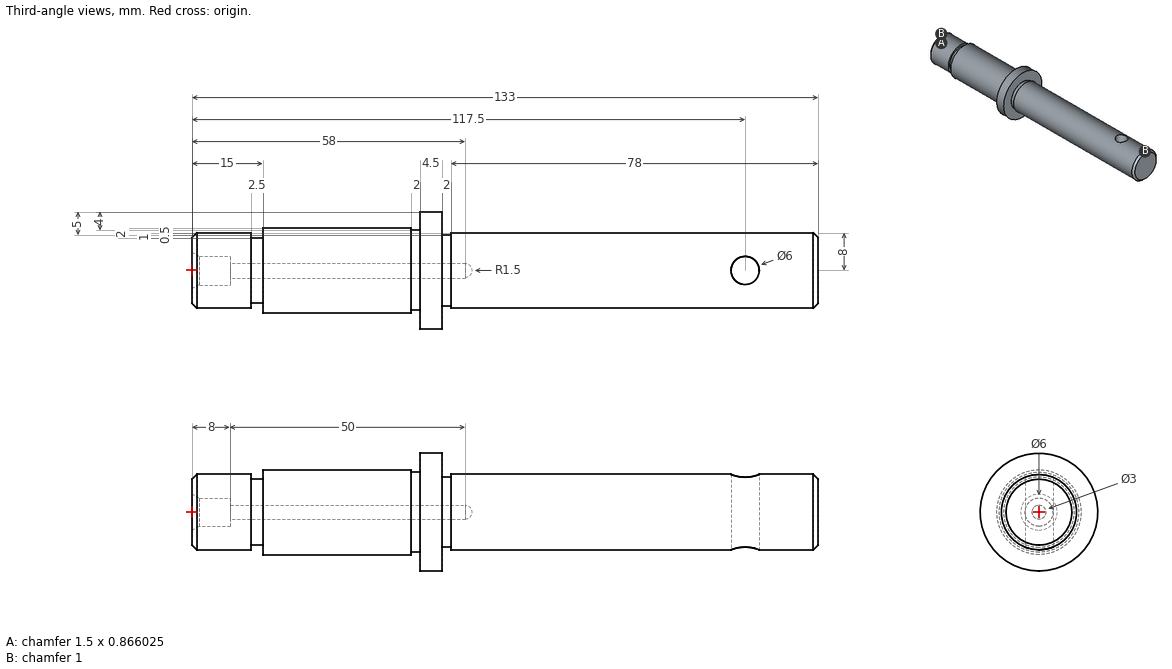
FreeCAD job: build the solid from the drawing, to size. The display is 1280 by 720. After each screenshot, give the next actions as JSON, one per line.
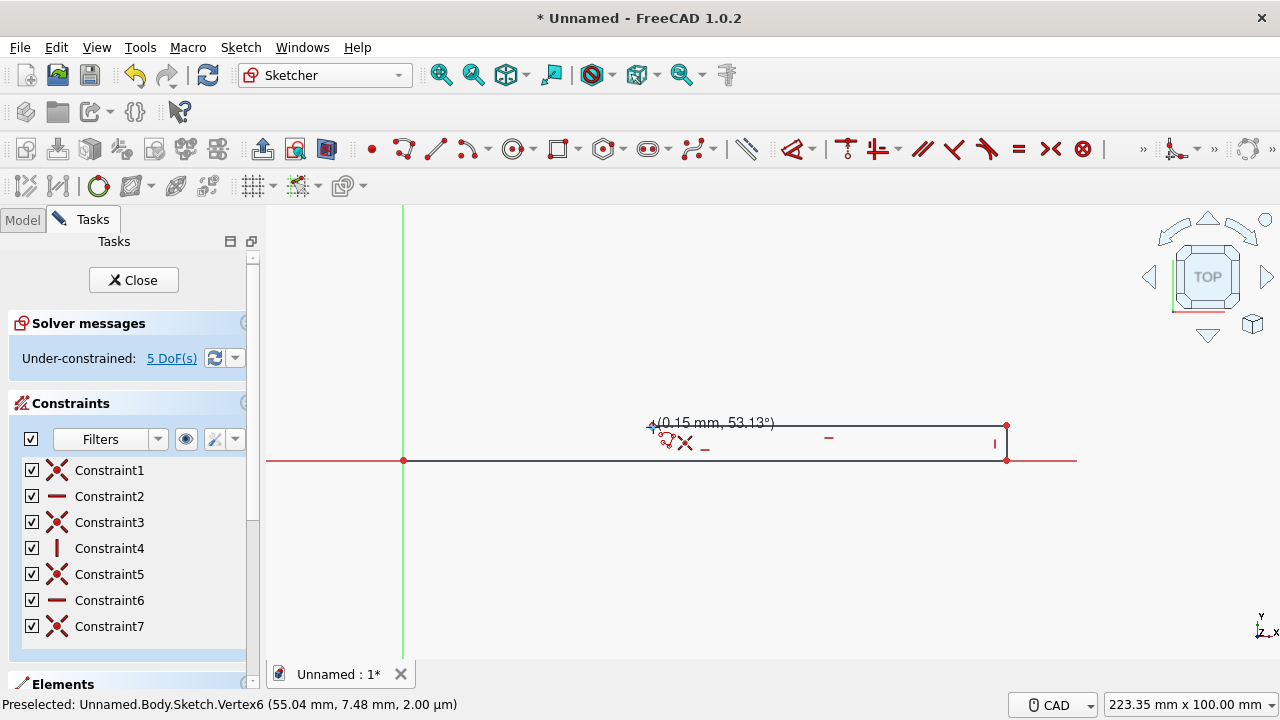
{"action": "scroll", "coordinate": [644, 427], "scroll_direction": "up", "scroll_amount": 3}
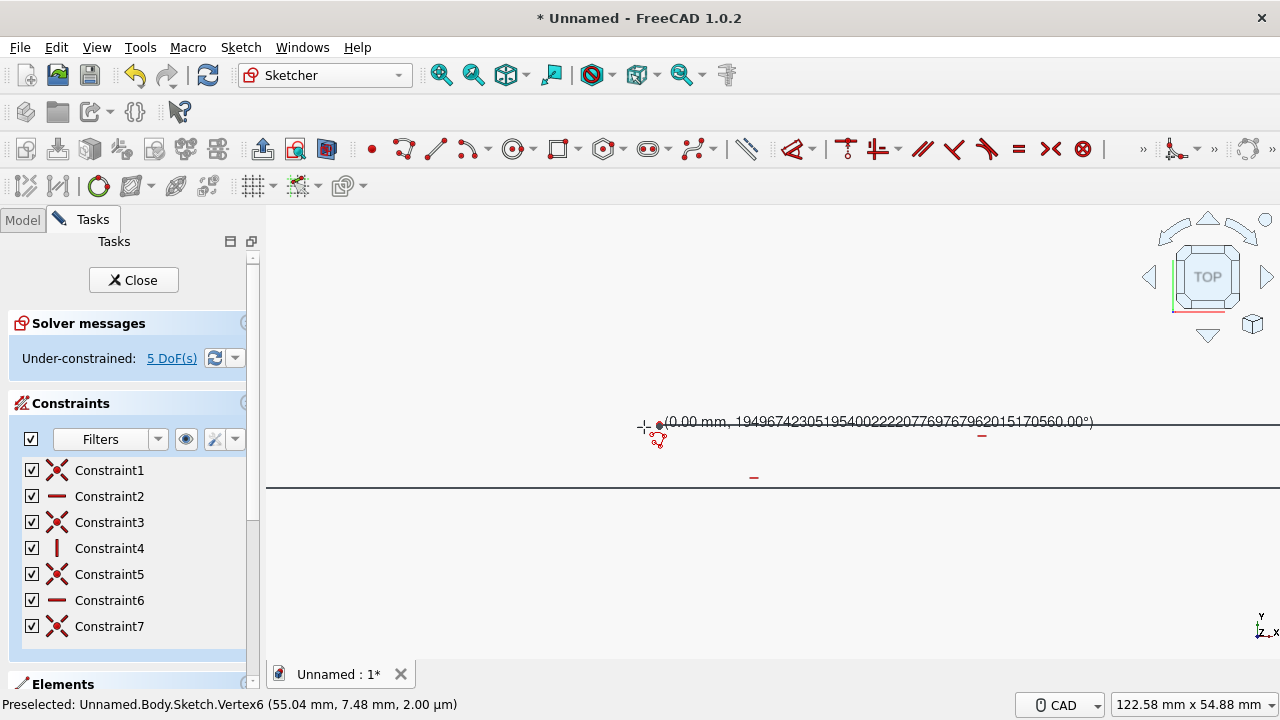
{"action": "left_click", "coordinate": [643, 426]}
{"action": "left_click", "coordinate": [643, 385]}
{"action": "left_click", "coordinate": [606, 385]}
{"action": "left_click", "coordinate": [606, 418]}
{"action": "left_click", "coordinate": [590, 418]}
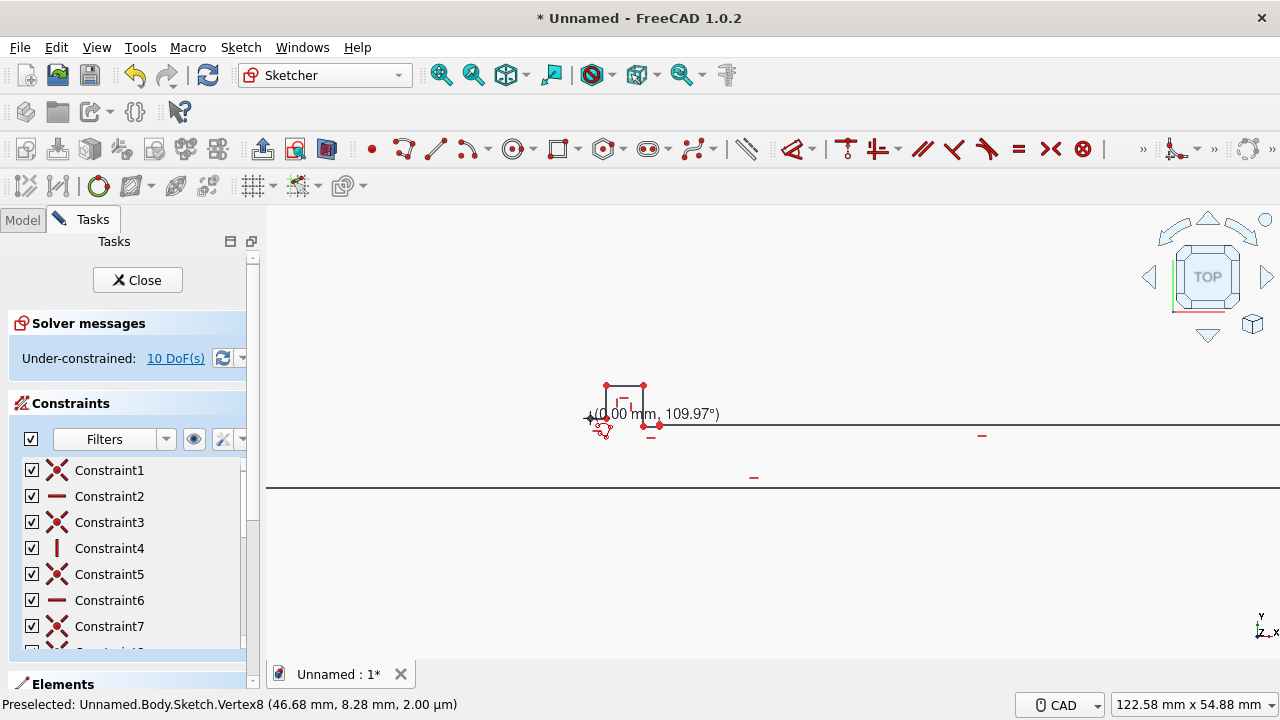
{"action": "scroll", "coordinate": [590, 414], "scroll_direction": "up", "scroll_amount": 7}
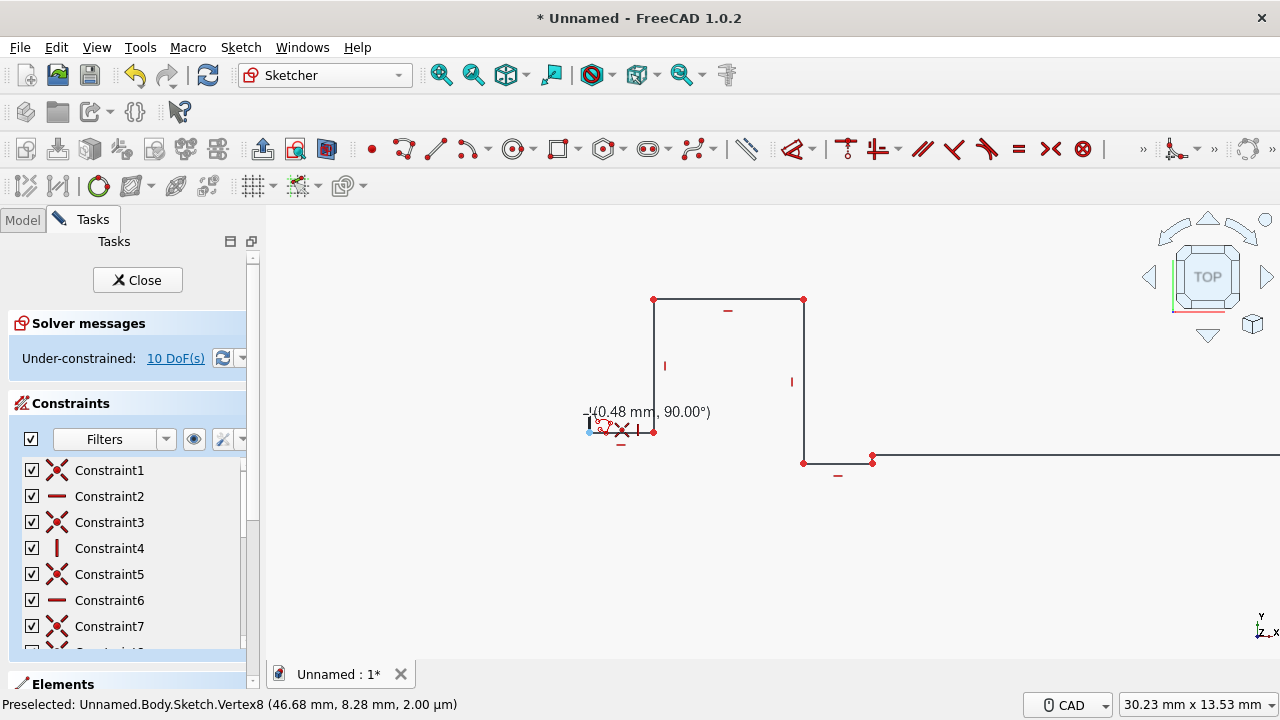
{"action": "left_click", "coordinate": [589, 413]}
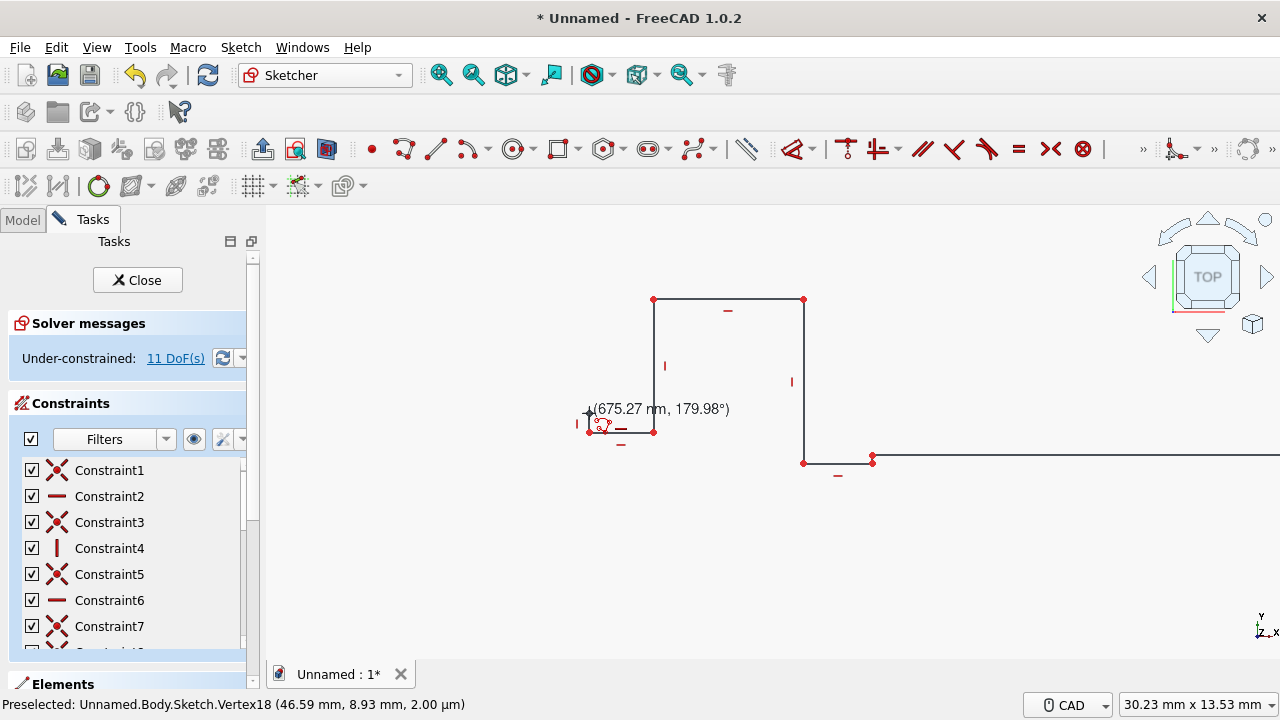
{"action": "scroll", "coordinate": [618, 421], "scroll_direction": "down", "scroll_amount": 10}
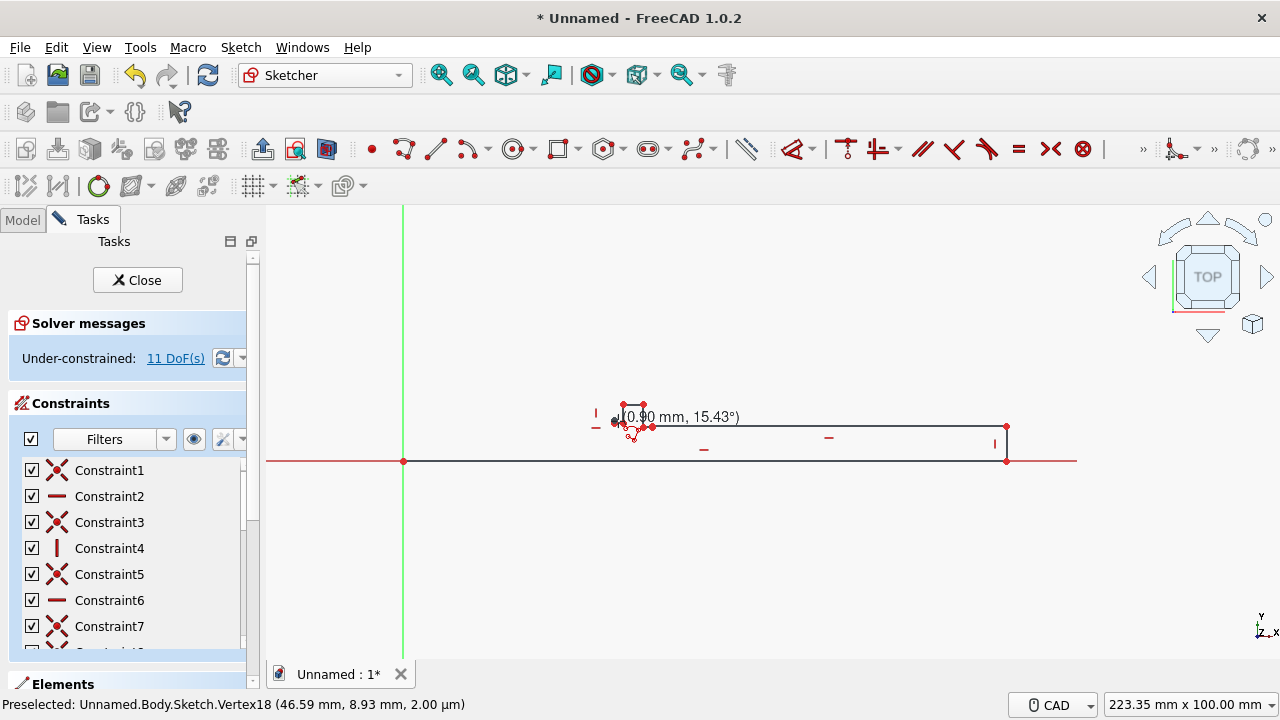
{"action": "left_click", "coordinate": [471, 420]}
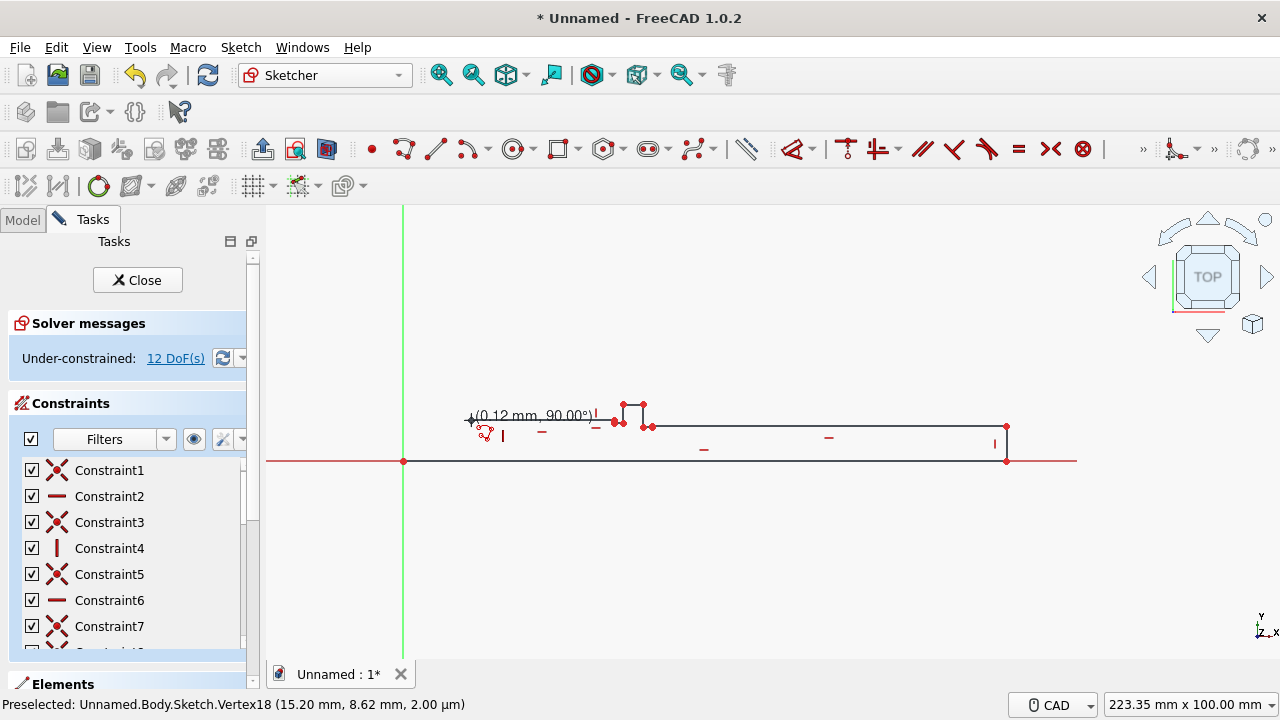
{"action": "scroll", "coordinate": [471, 429], "scroll_direction": "up", "scroll_amount": 3}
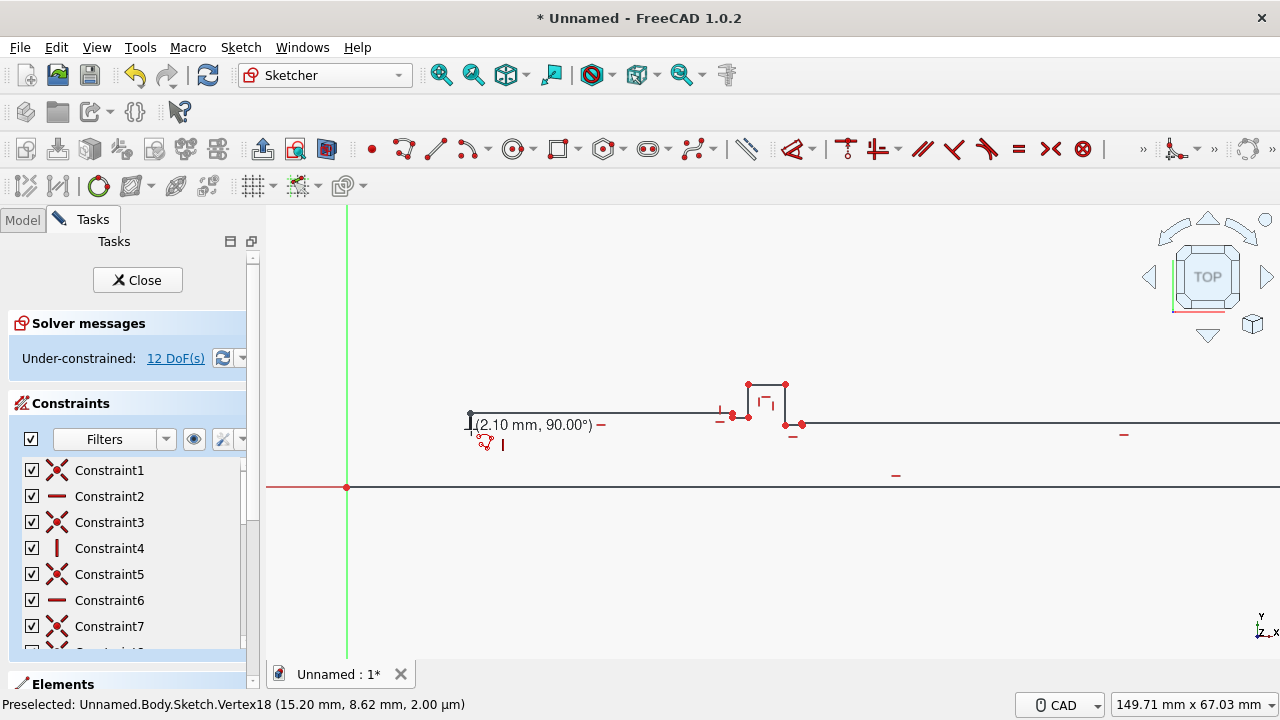
{"action": "left_click", "coordinate": [471, 429]}
{"action": "left_click", "coordinate": [450, 429]}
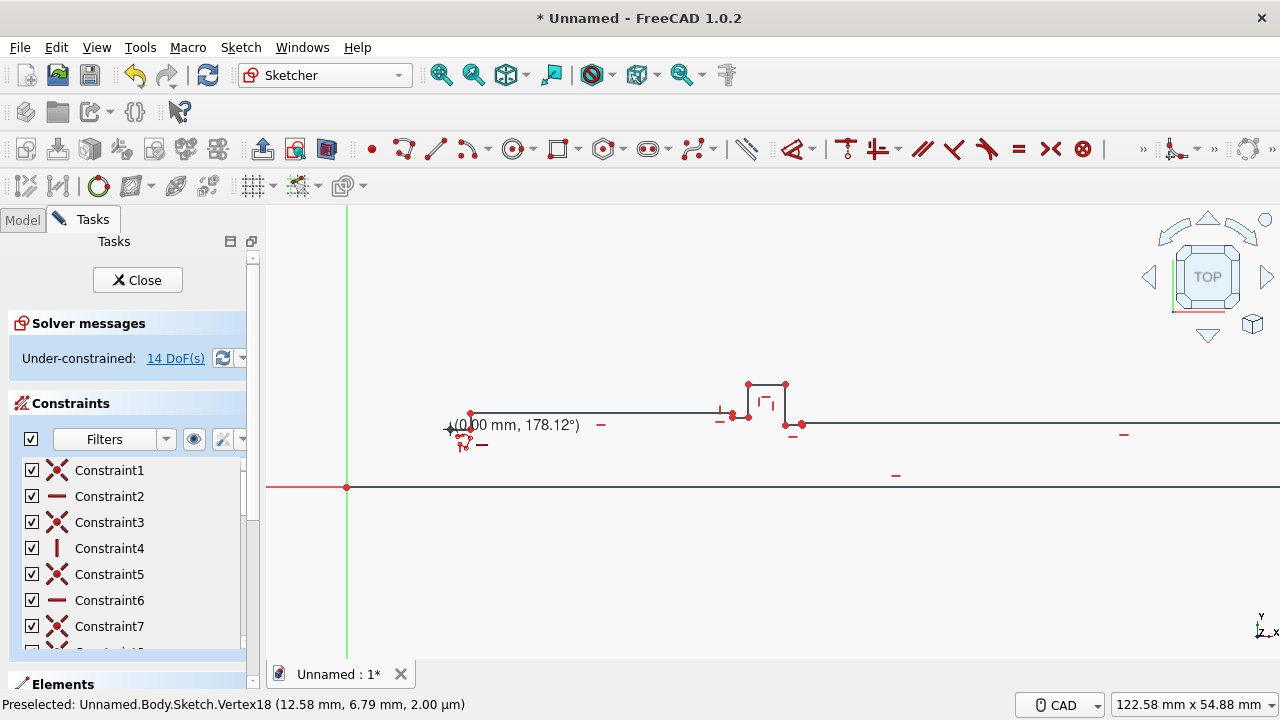
{"action": "scroll", "coordinate": [450, 421], "scroll_direction": "up", "scroll_amount": 4}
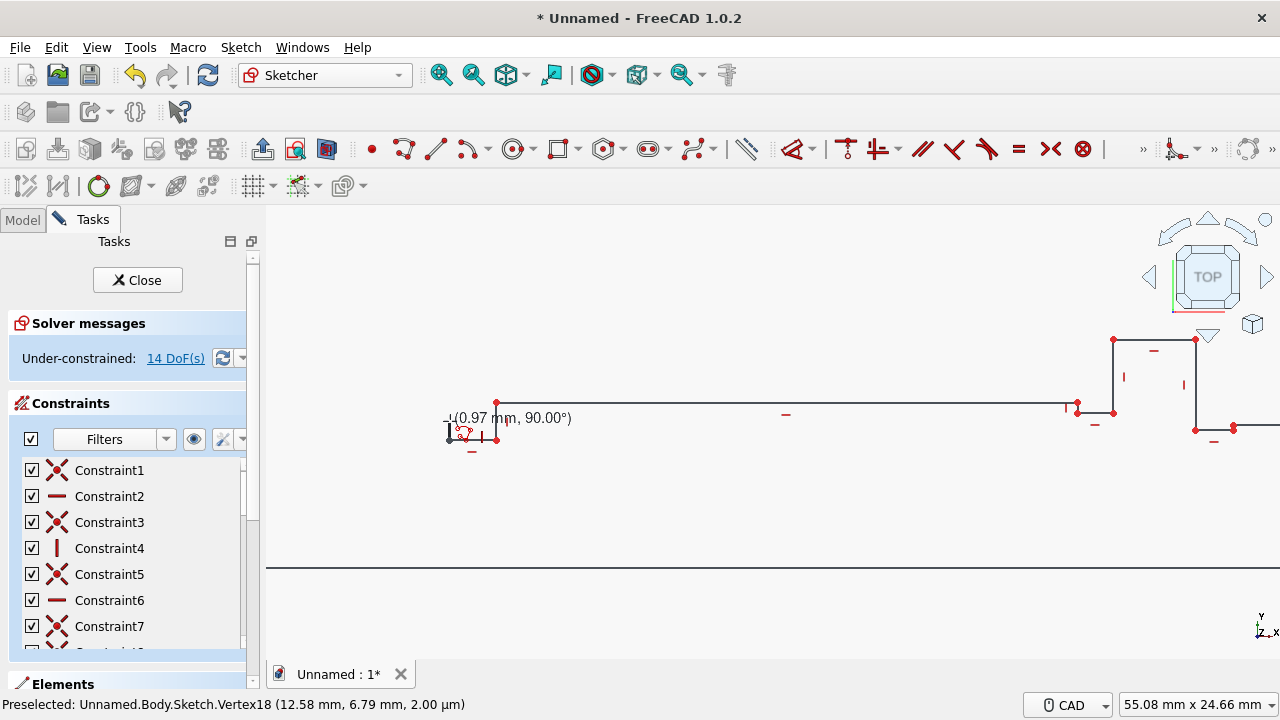
{"action": "left_click", "coordinate": [450, 420]}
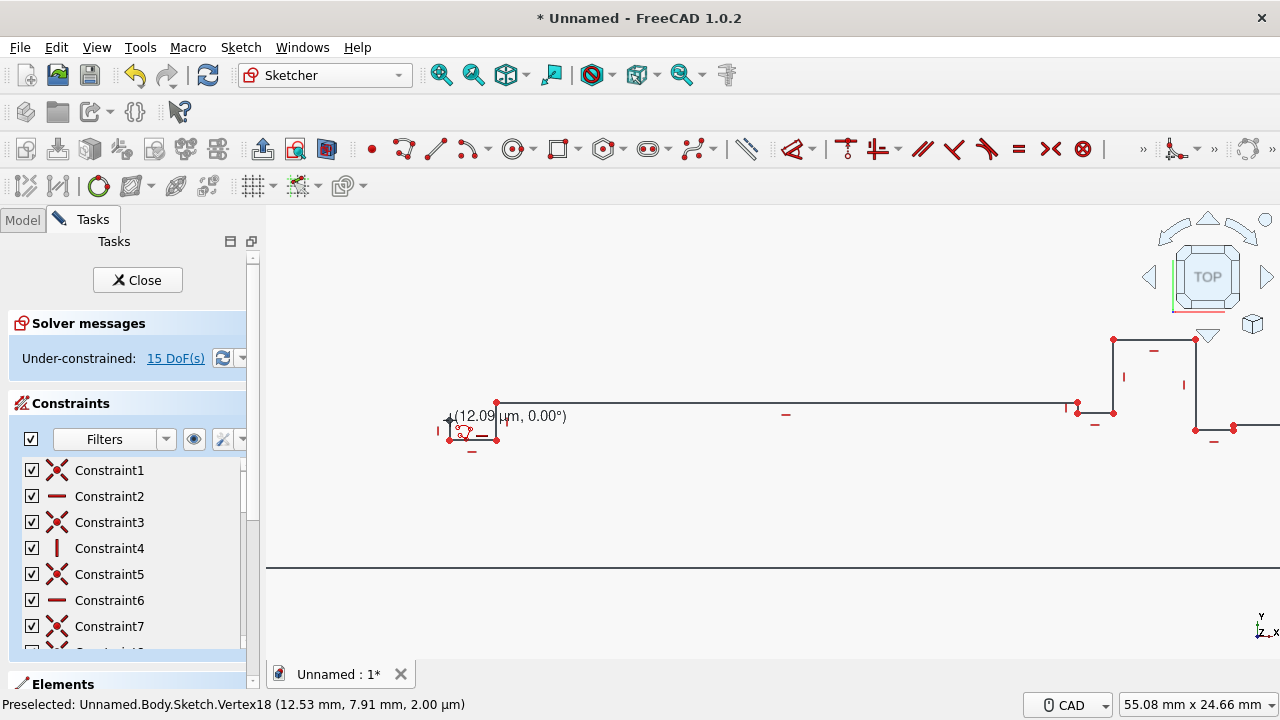
{"action": "scroll", "coordinate": [462, 425], "scroll_direction": "down", "scroll_amount": 7}